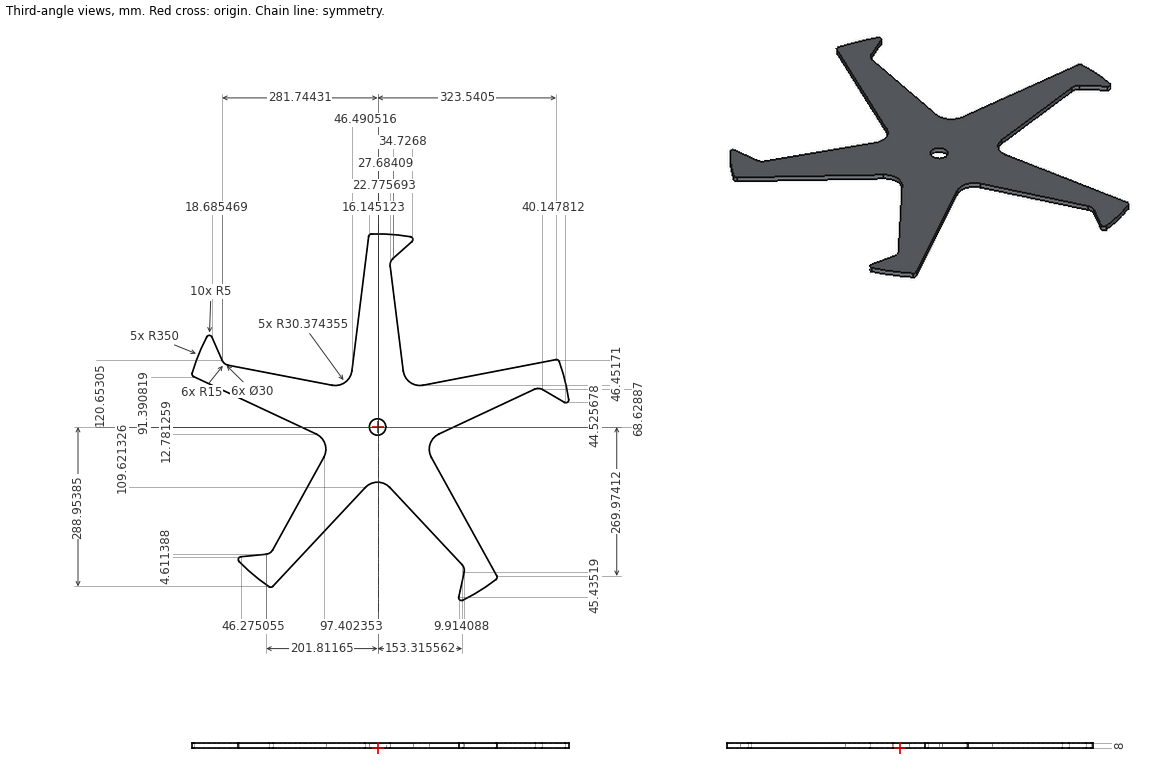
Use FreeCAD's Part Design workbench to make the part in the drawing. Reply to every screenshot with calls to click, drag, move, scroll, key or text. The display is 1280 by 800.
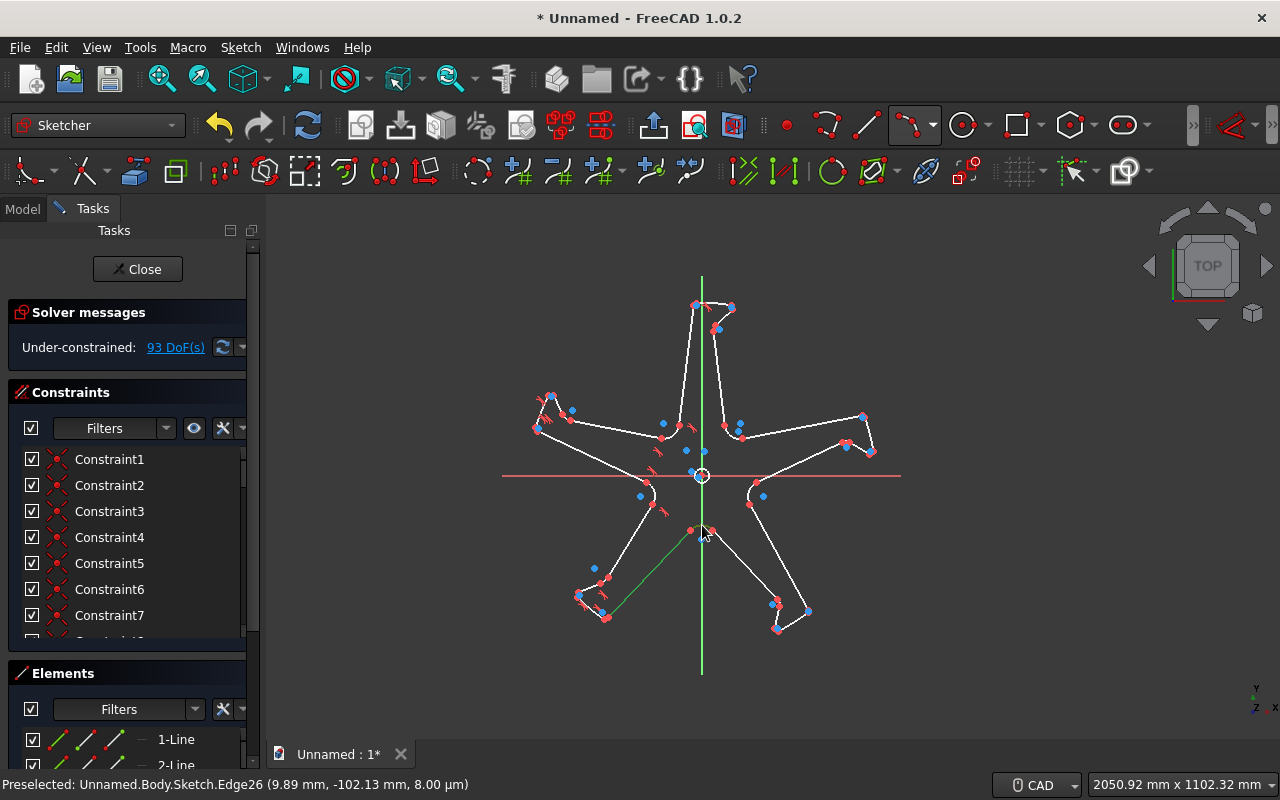
key(t)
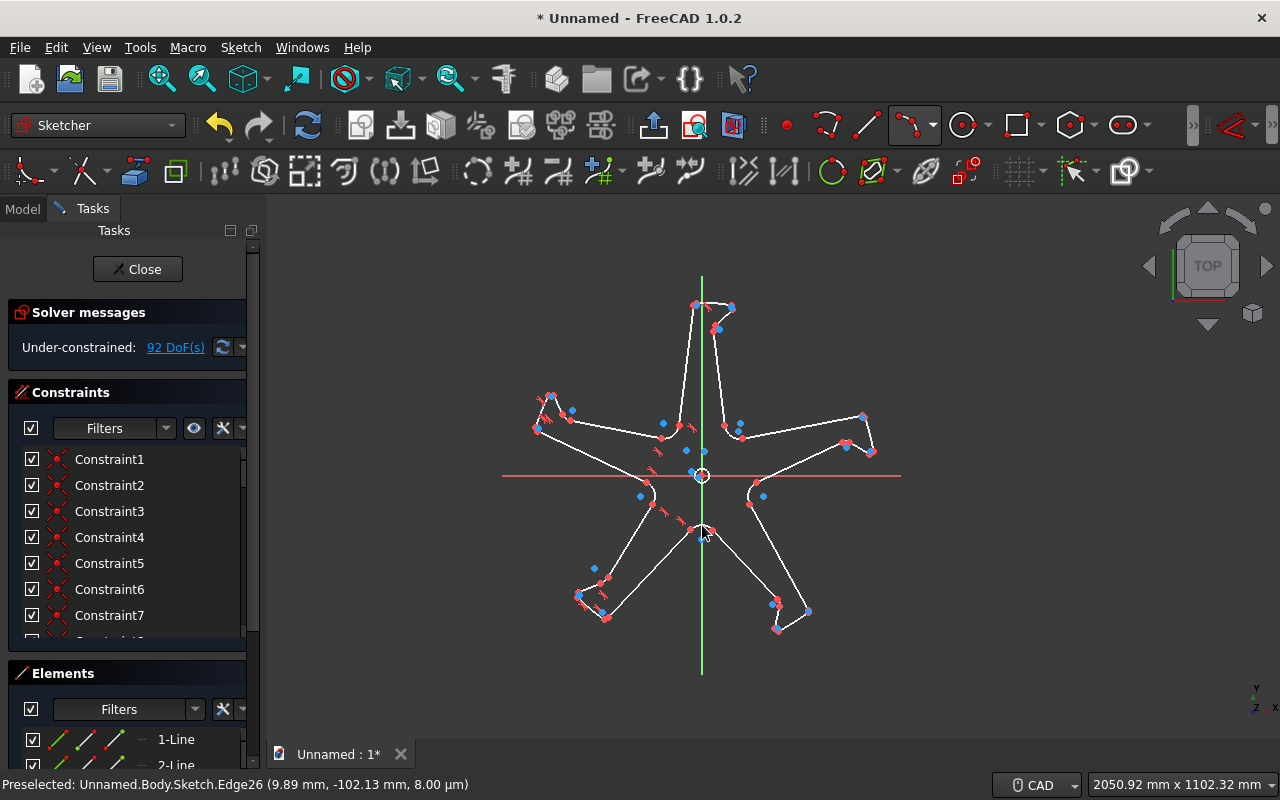
click(732, 551)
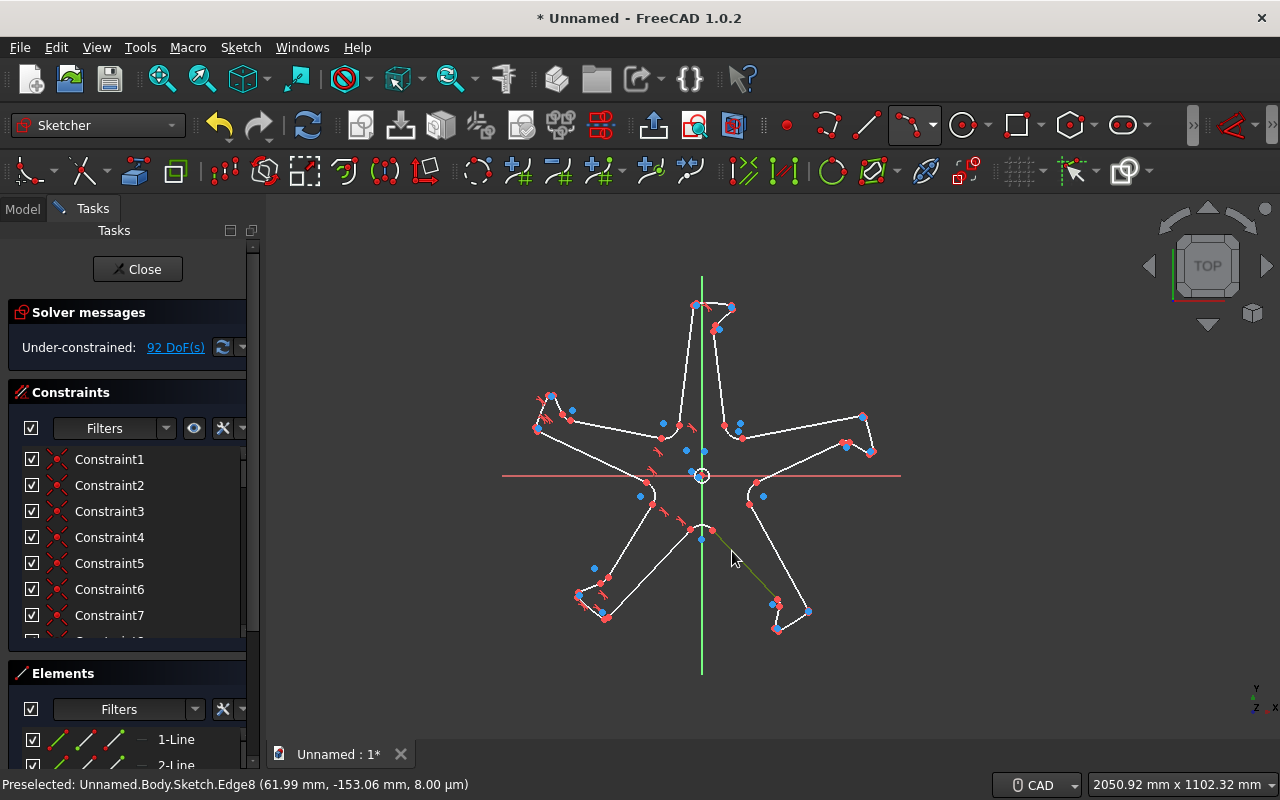
click(702, 525)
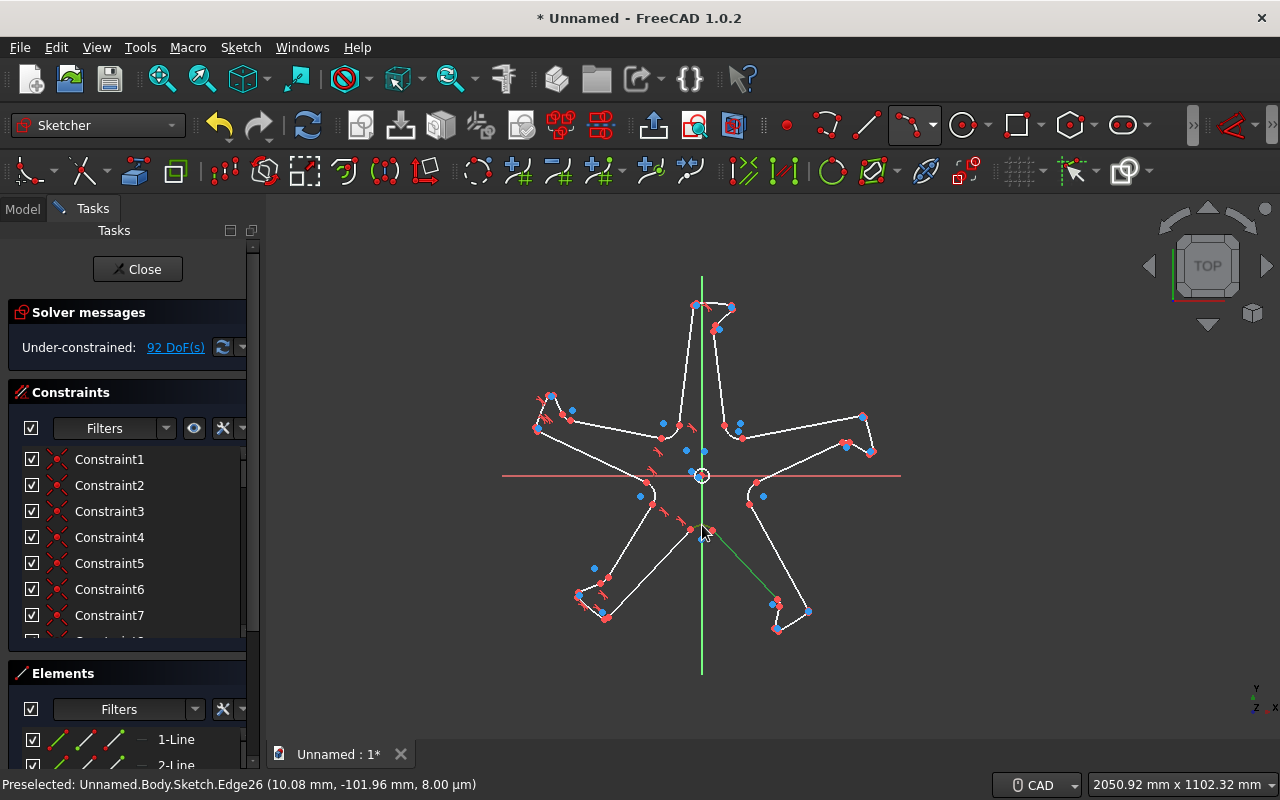
key(t)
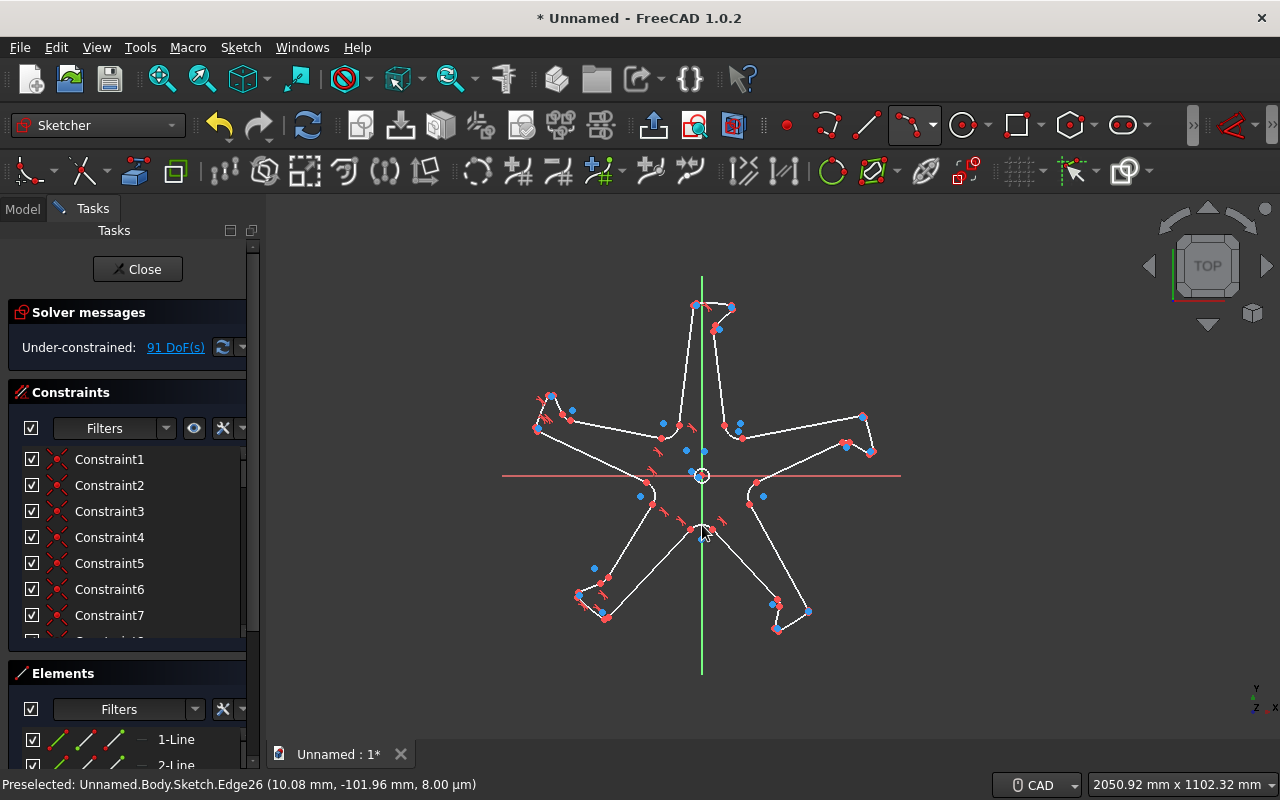
click(732, 551)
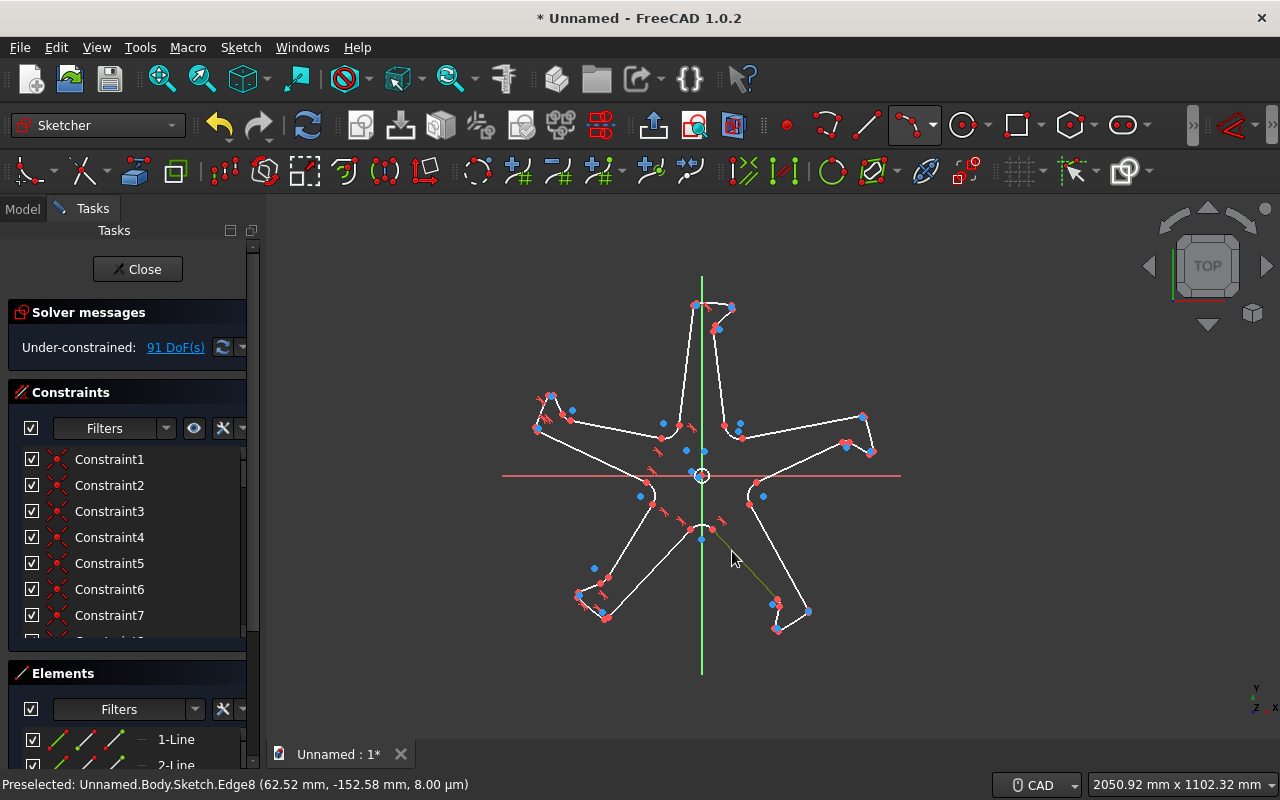
scroll(780, 603, up, 7)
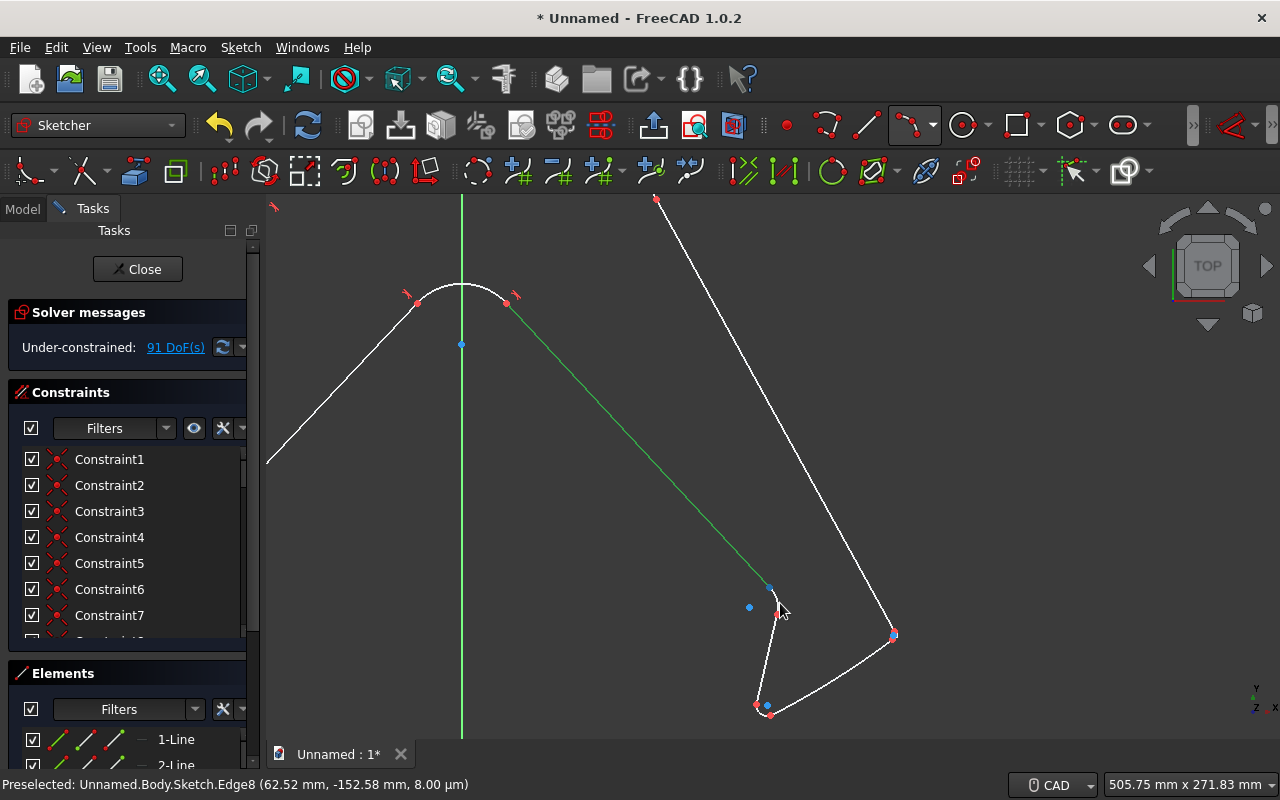
click(777, 600)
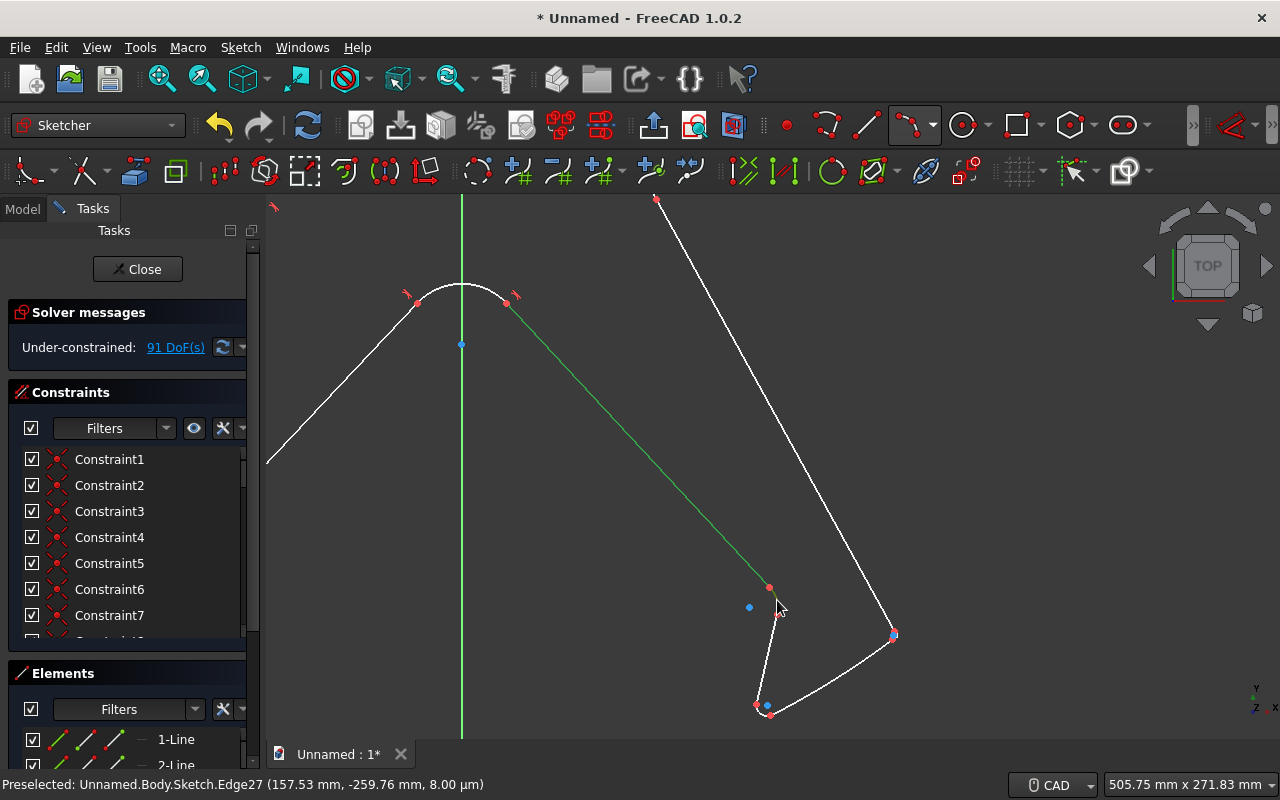
key(t)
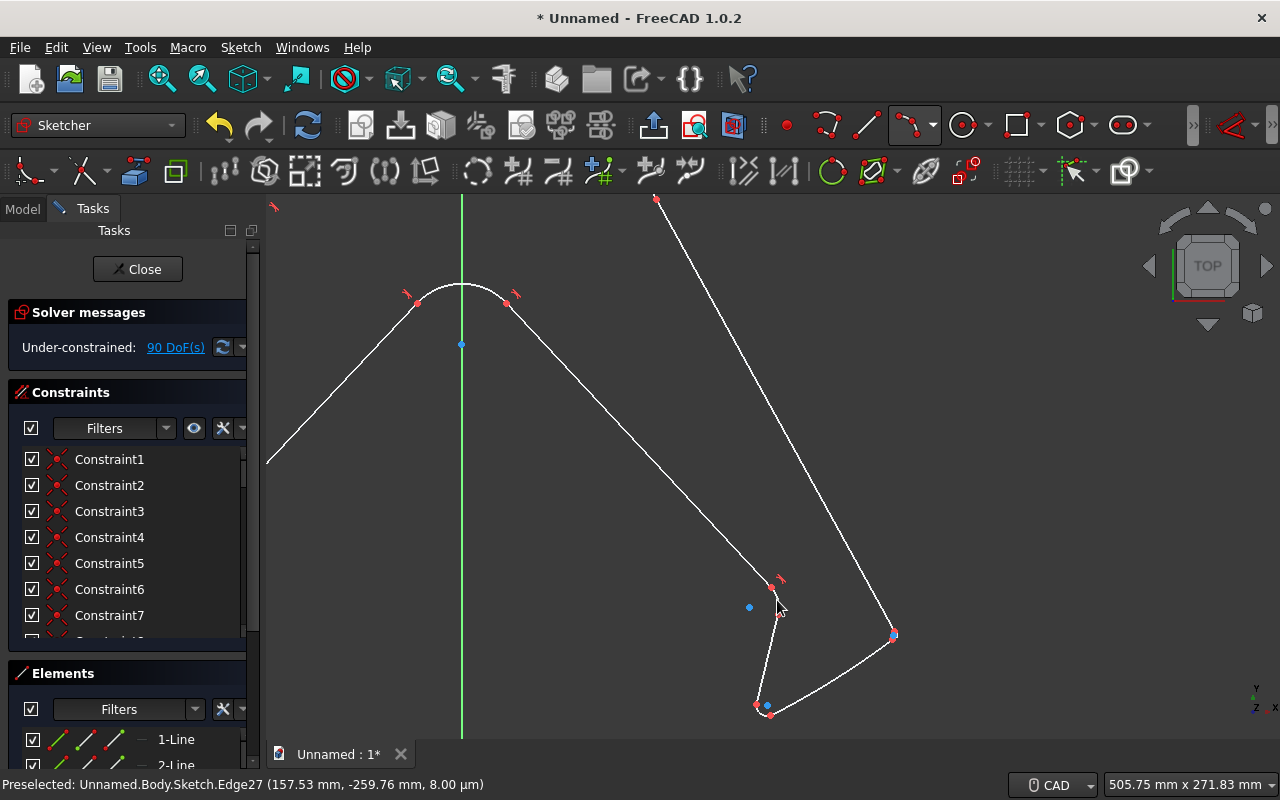
click(772, 641)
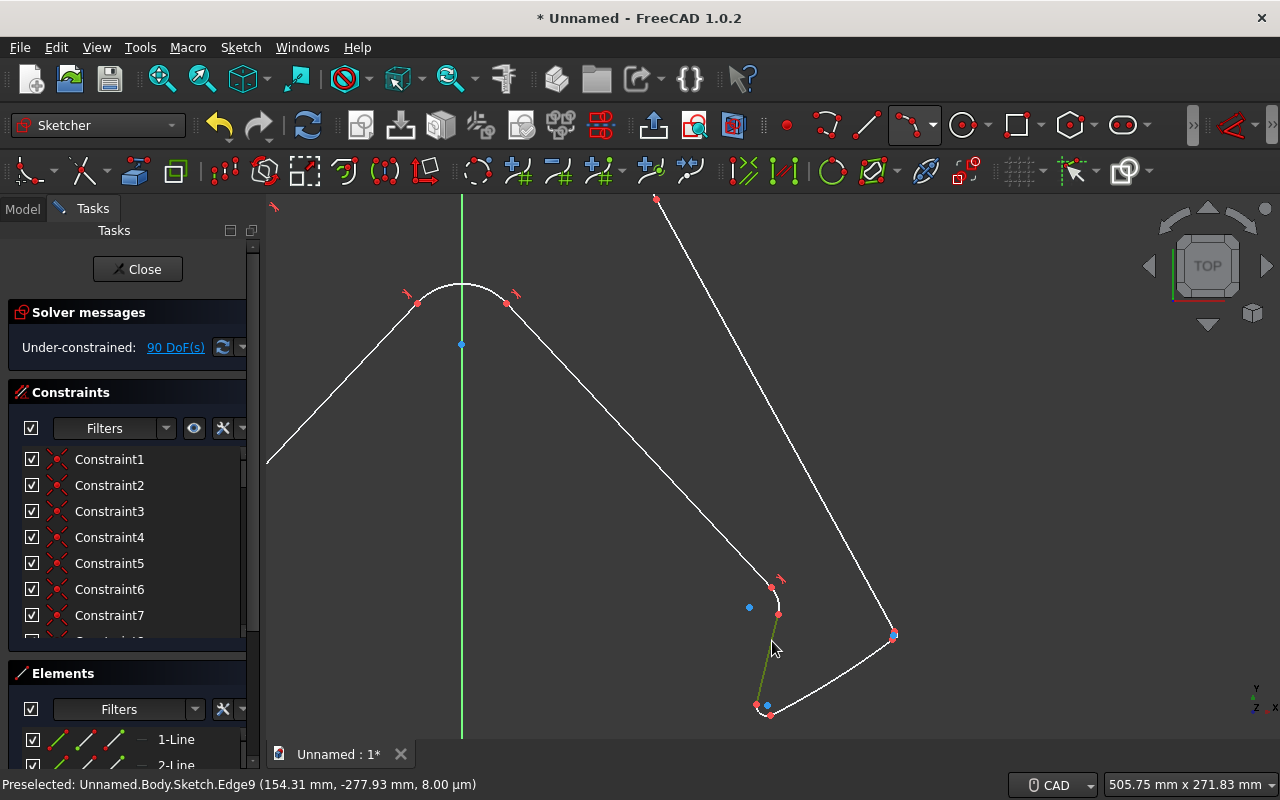
click(778, 600)